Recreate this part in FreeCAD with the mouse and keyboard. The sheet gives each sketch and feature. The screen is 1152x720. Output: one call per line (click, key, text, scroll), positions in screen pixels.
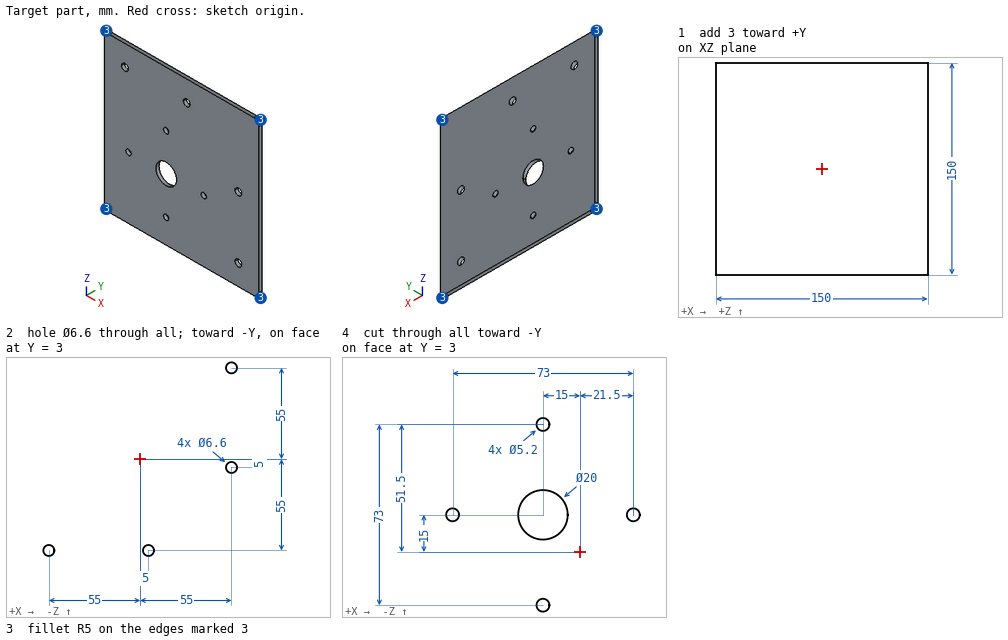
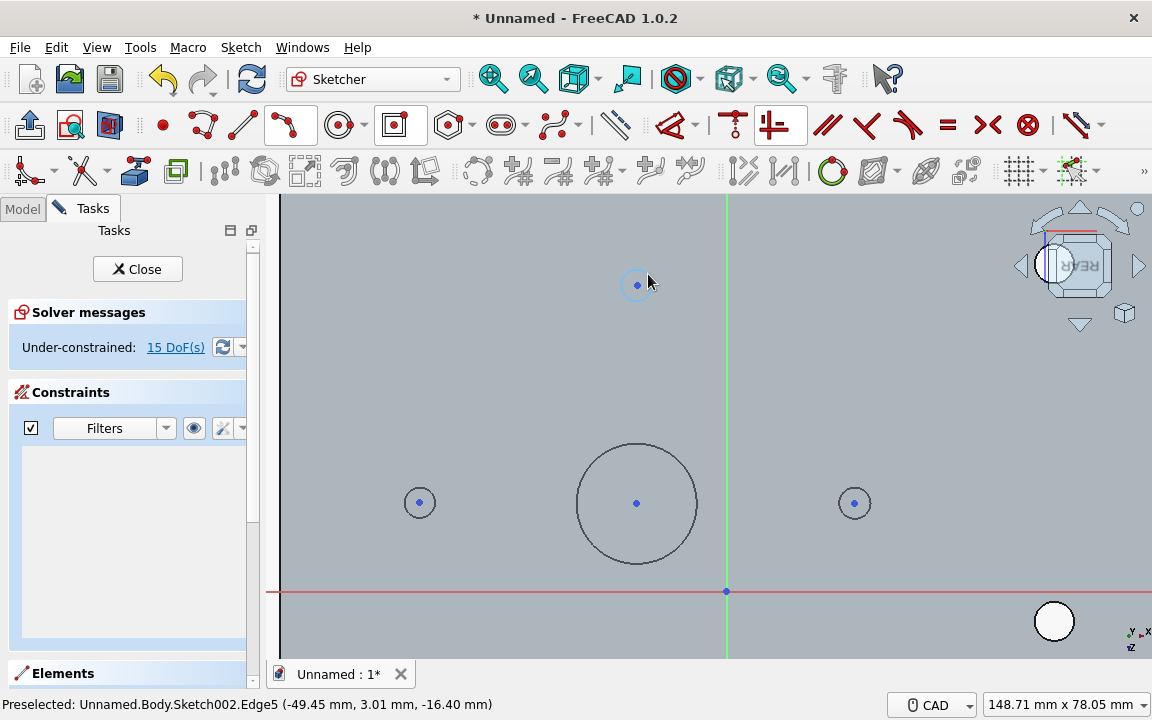
click(648, 274)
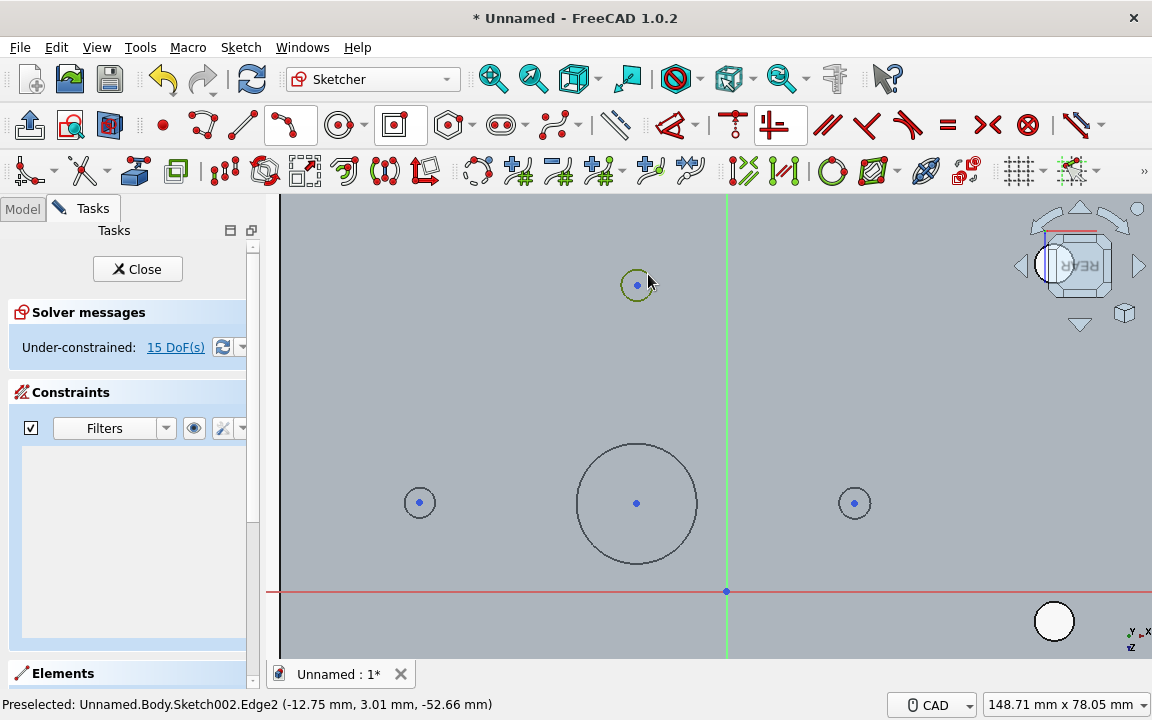
click(866, 492)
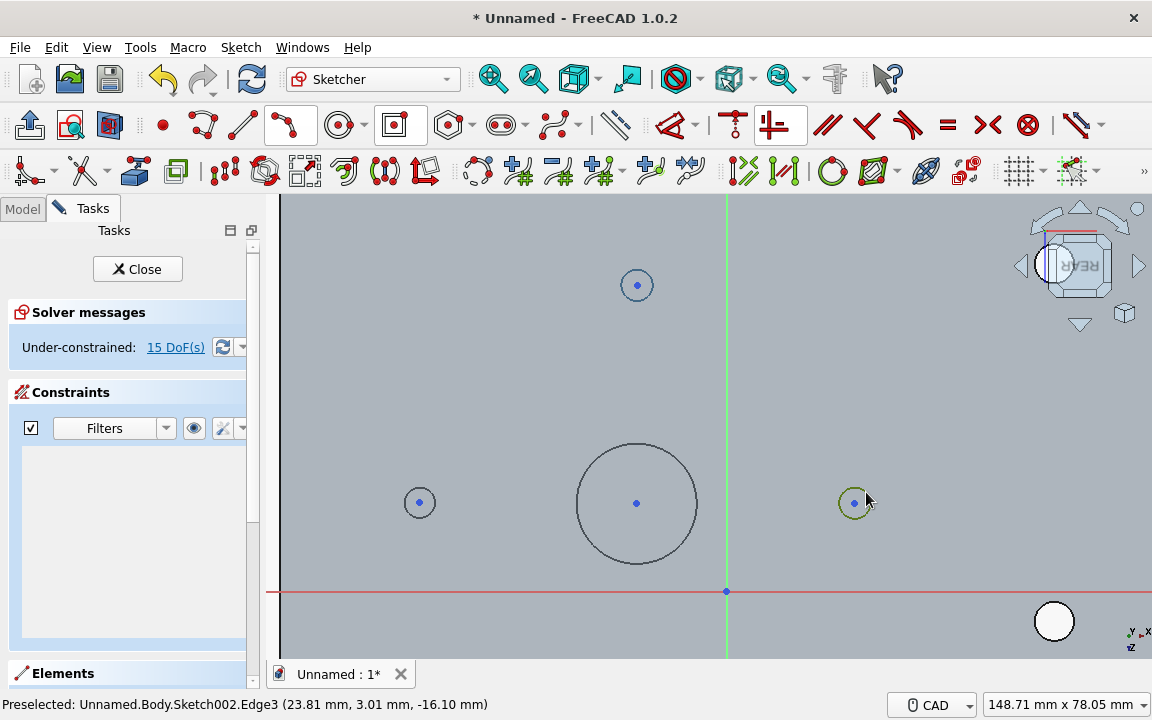
scroll(647, 273, down, 2)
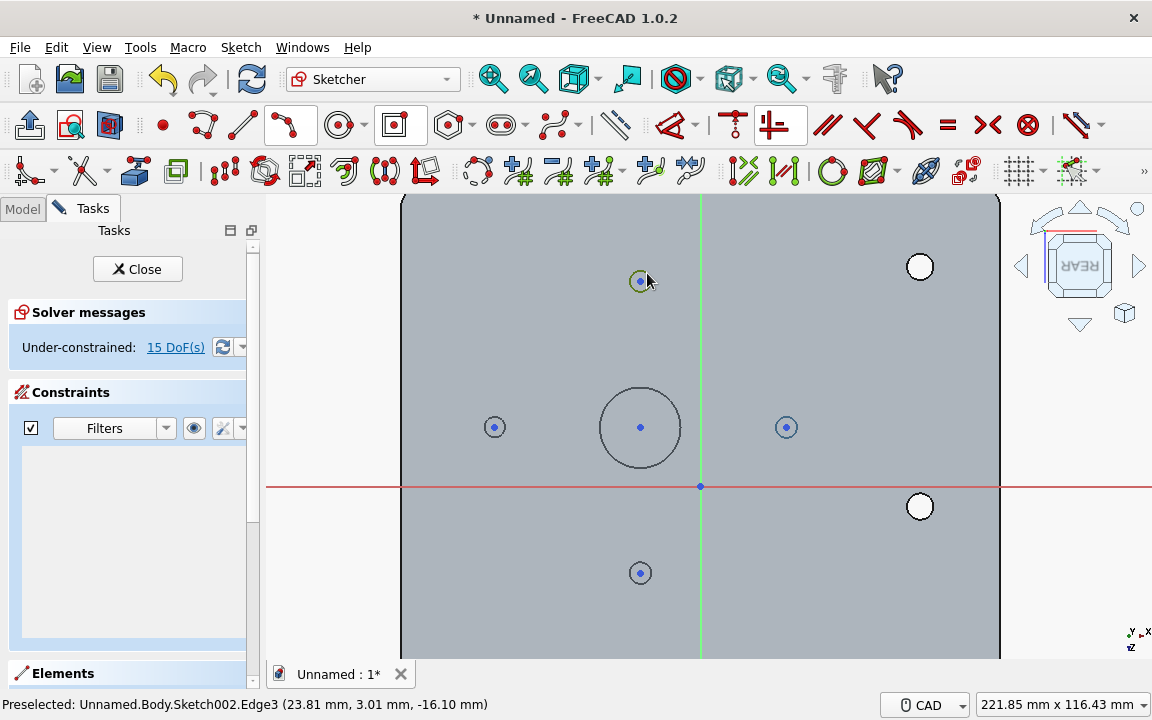
scroll(648, 565, up, 2)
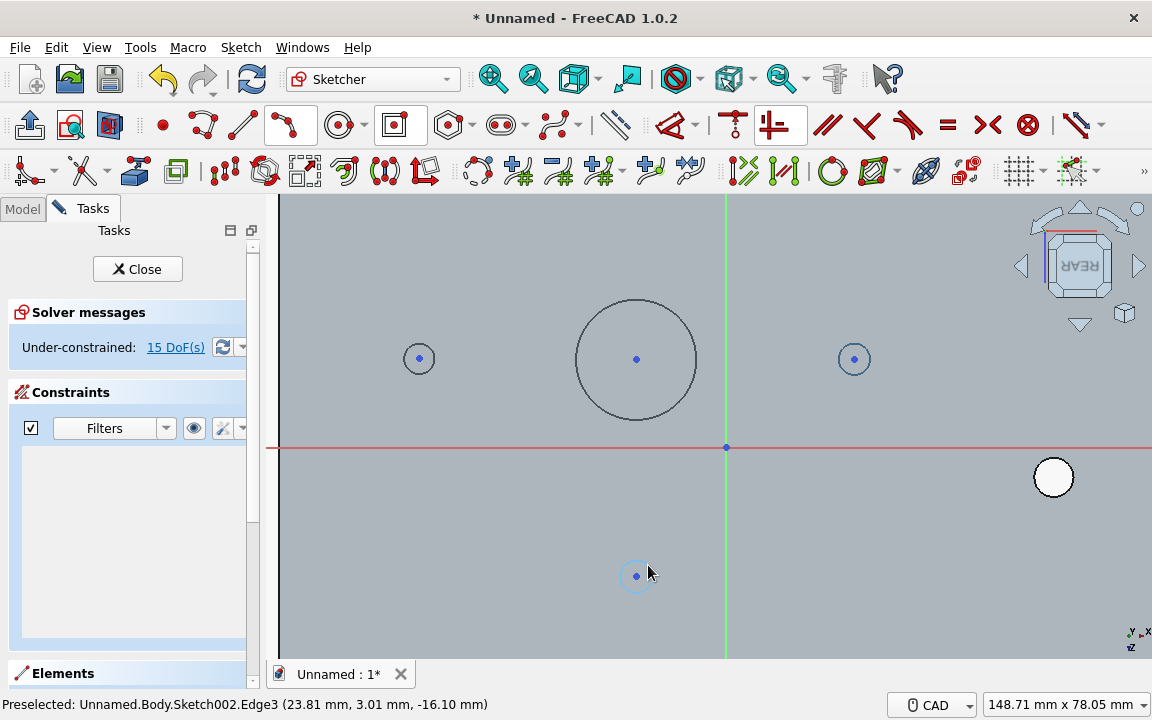
click(648, 565)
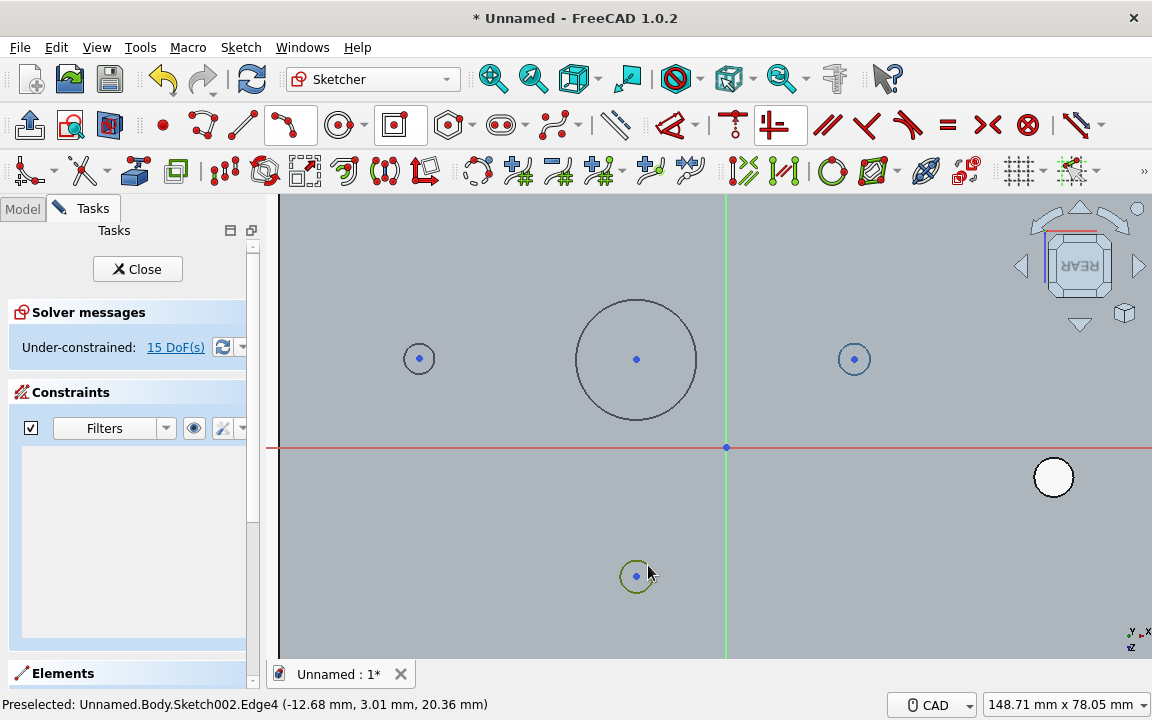
click(430, 348)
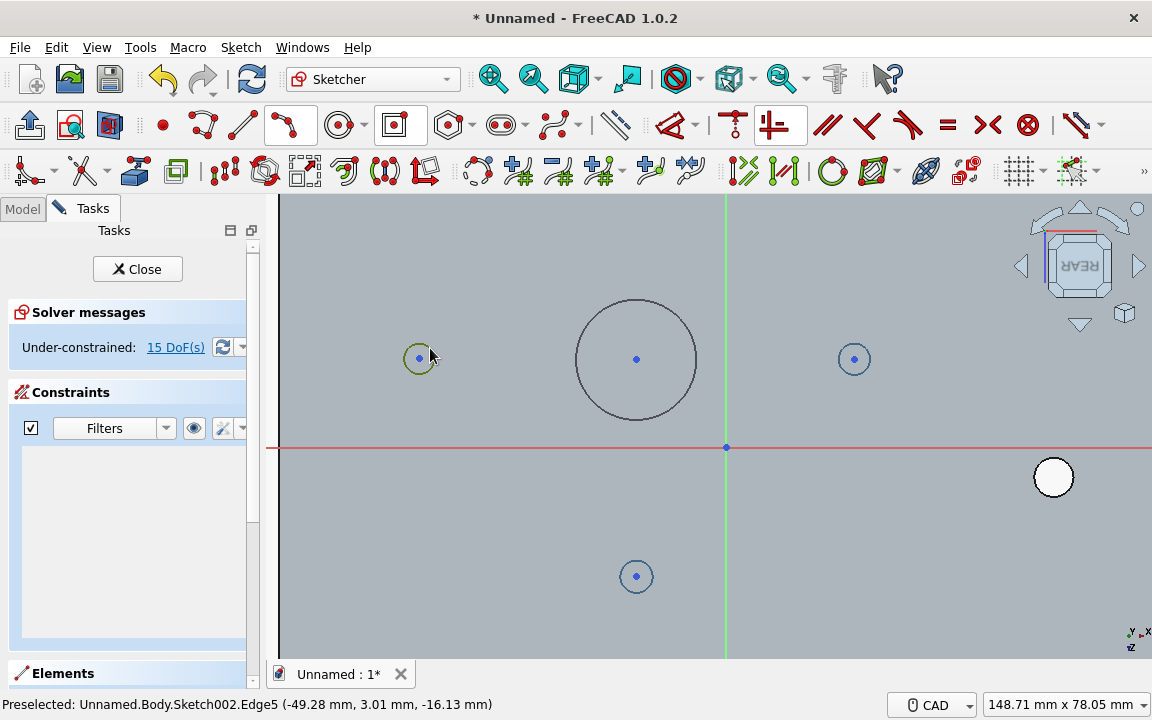
click(948, 126)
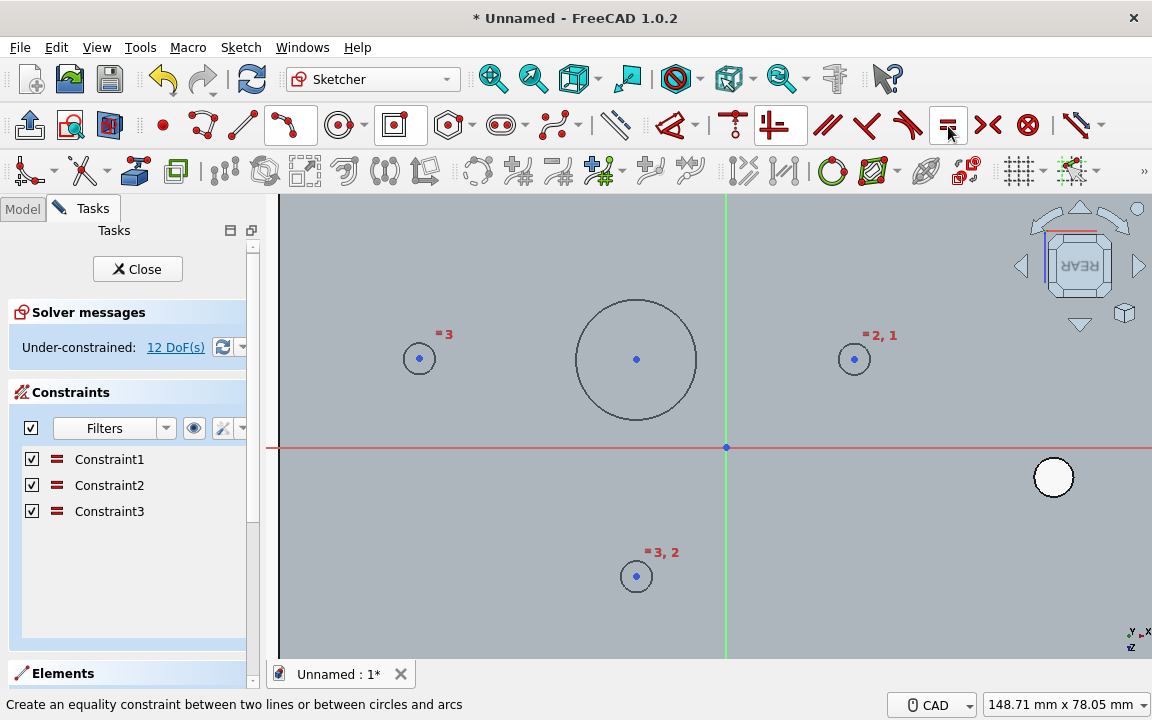
click(636, 360)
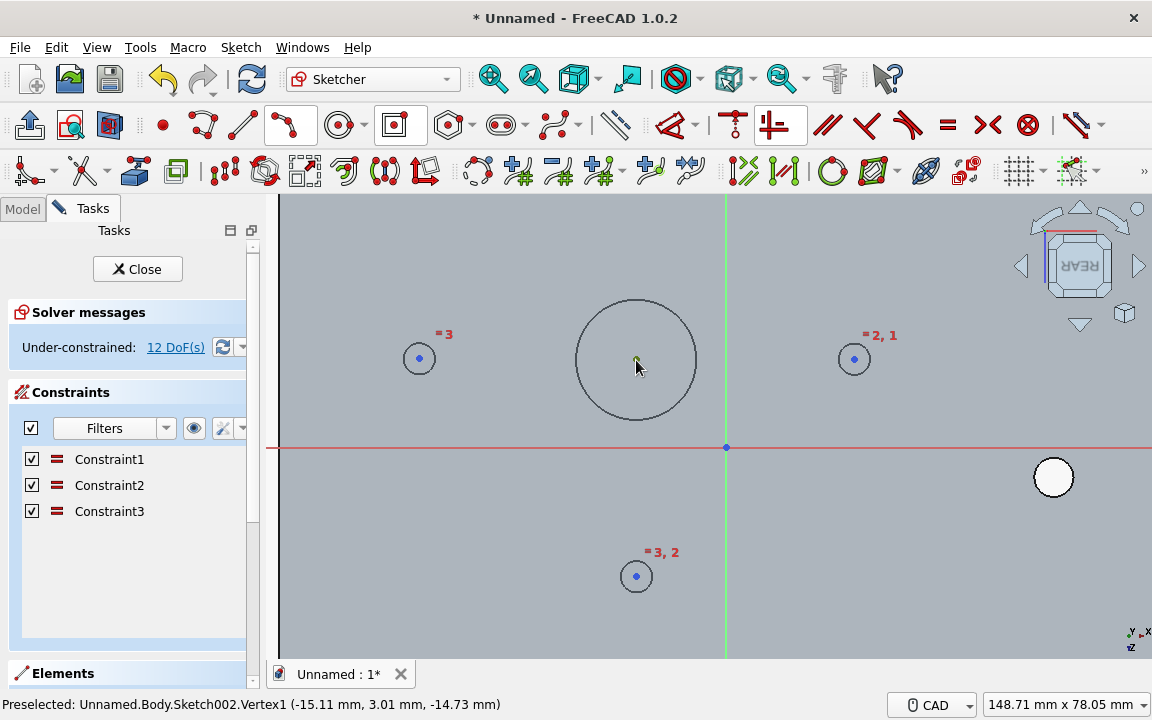
scroll(648, 565, down, 2)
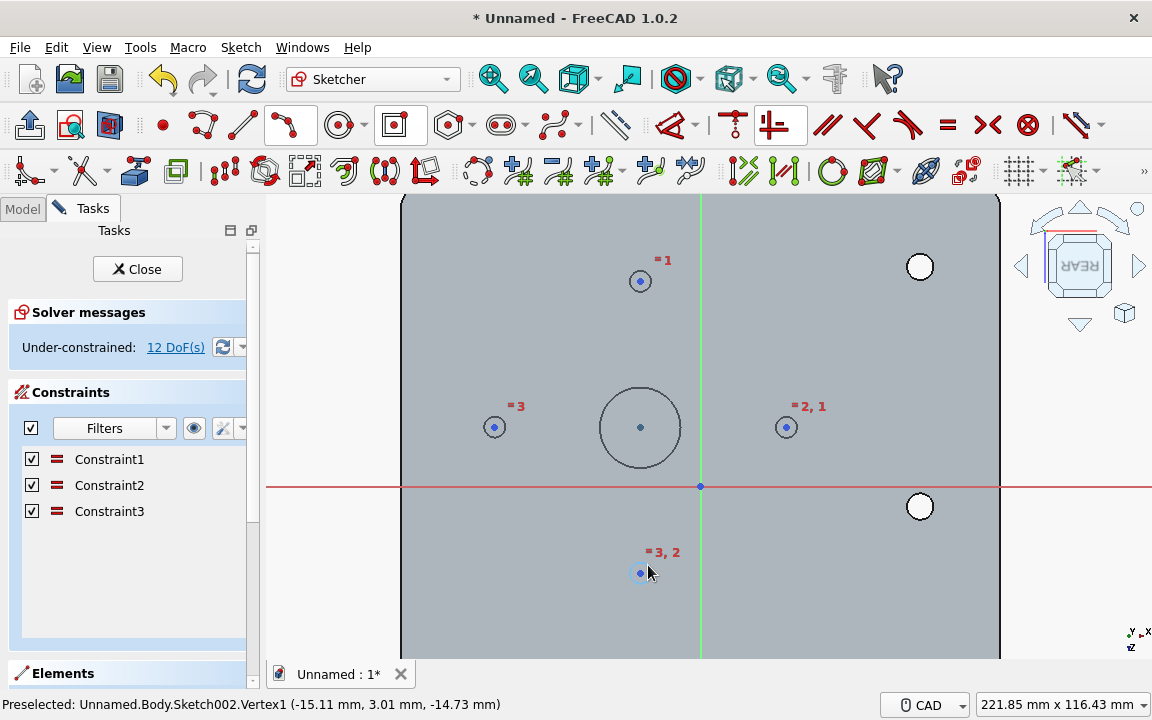
click(640, 281)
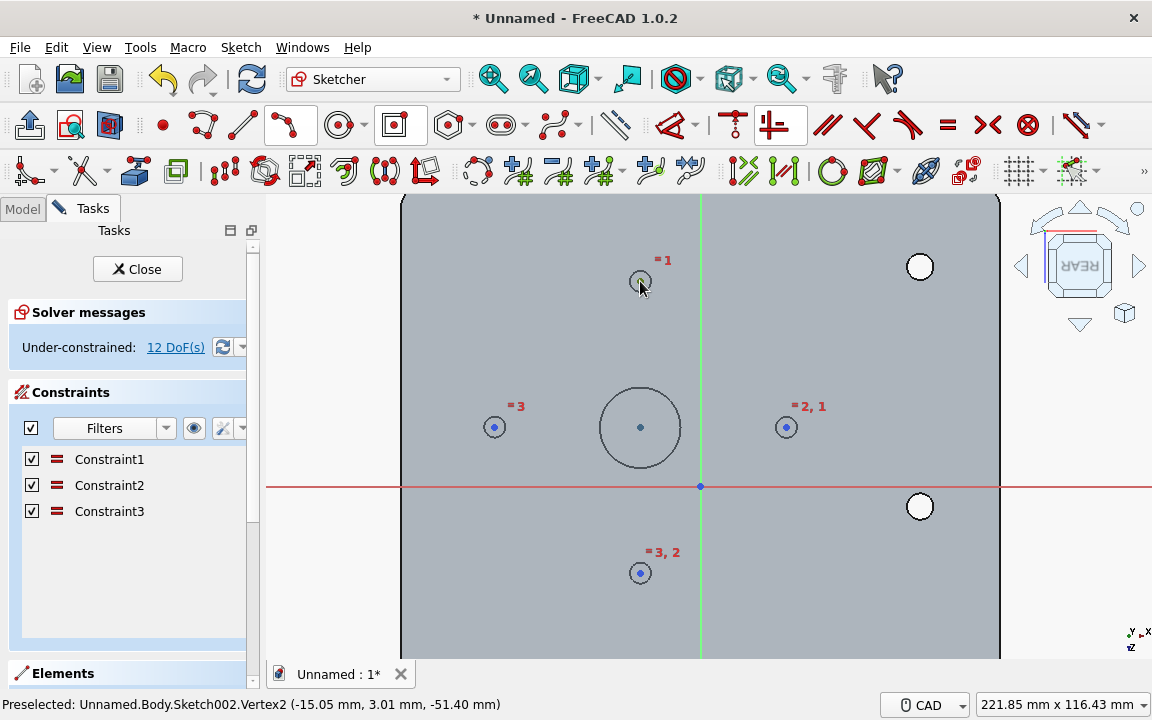
click(802, 126)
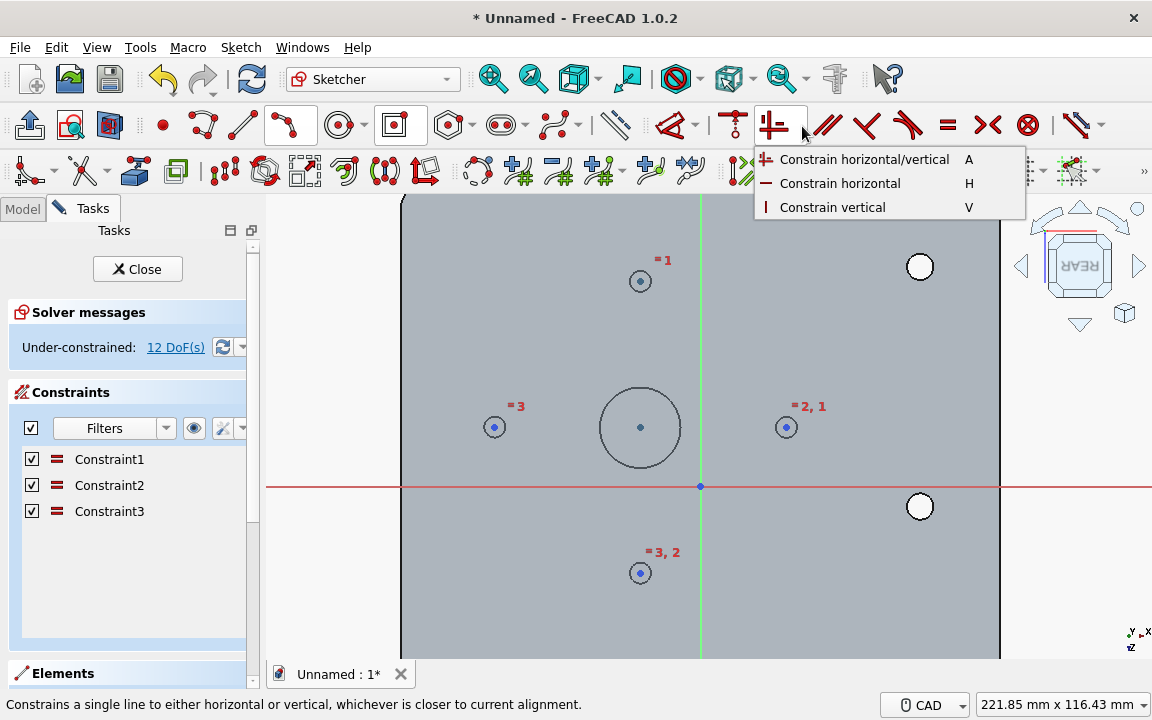
click(890, 207)